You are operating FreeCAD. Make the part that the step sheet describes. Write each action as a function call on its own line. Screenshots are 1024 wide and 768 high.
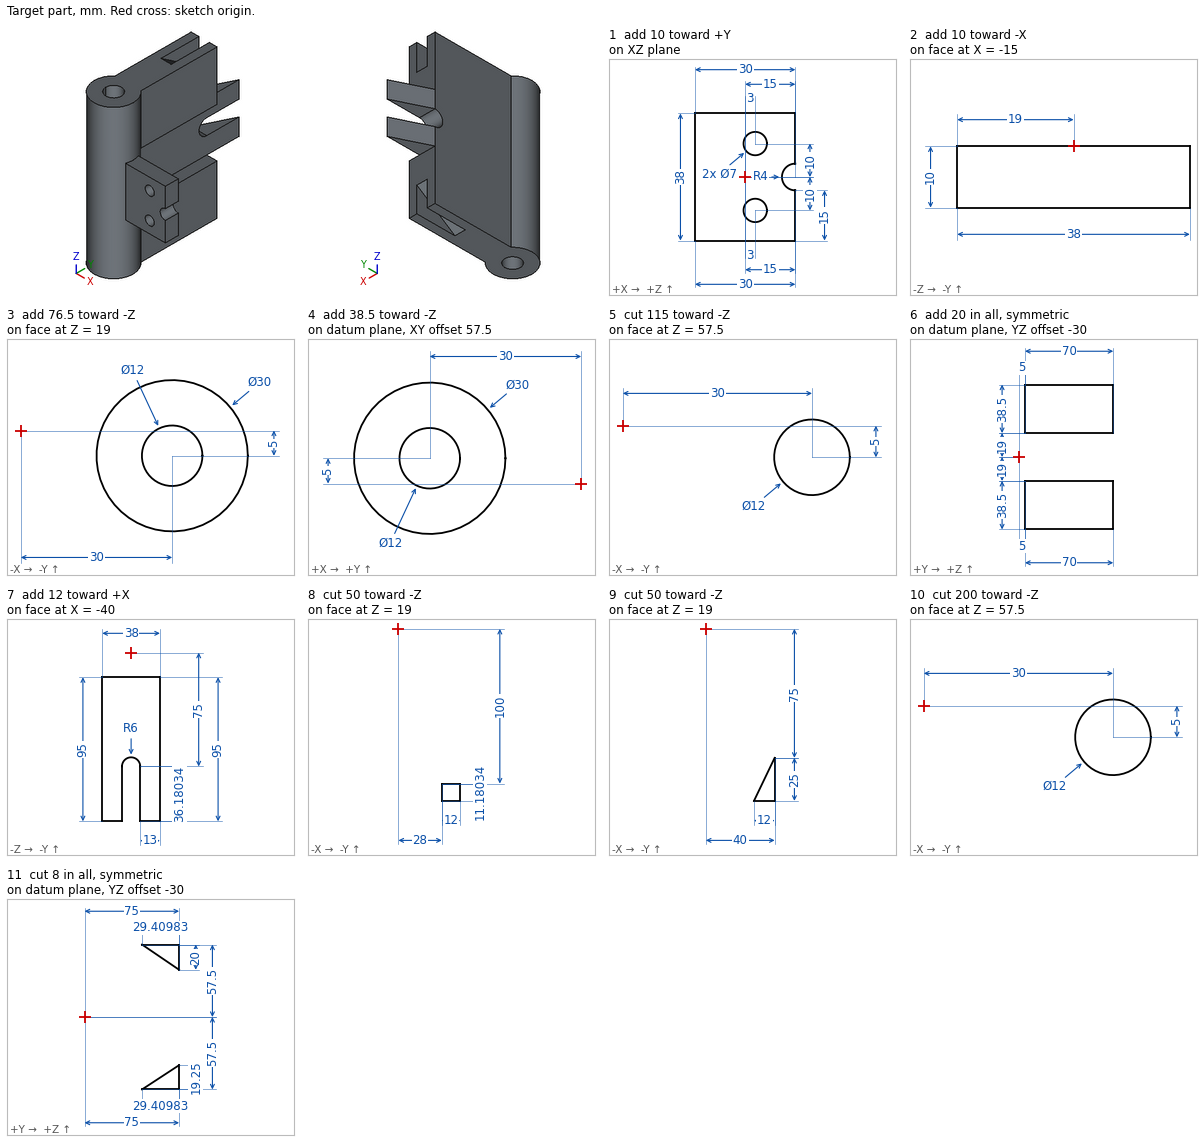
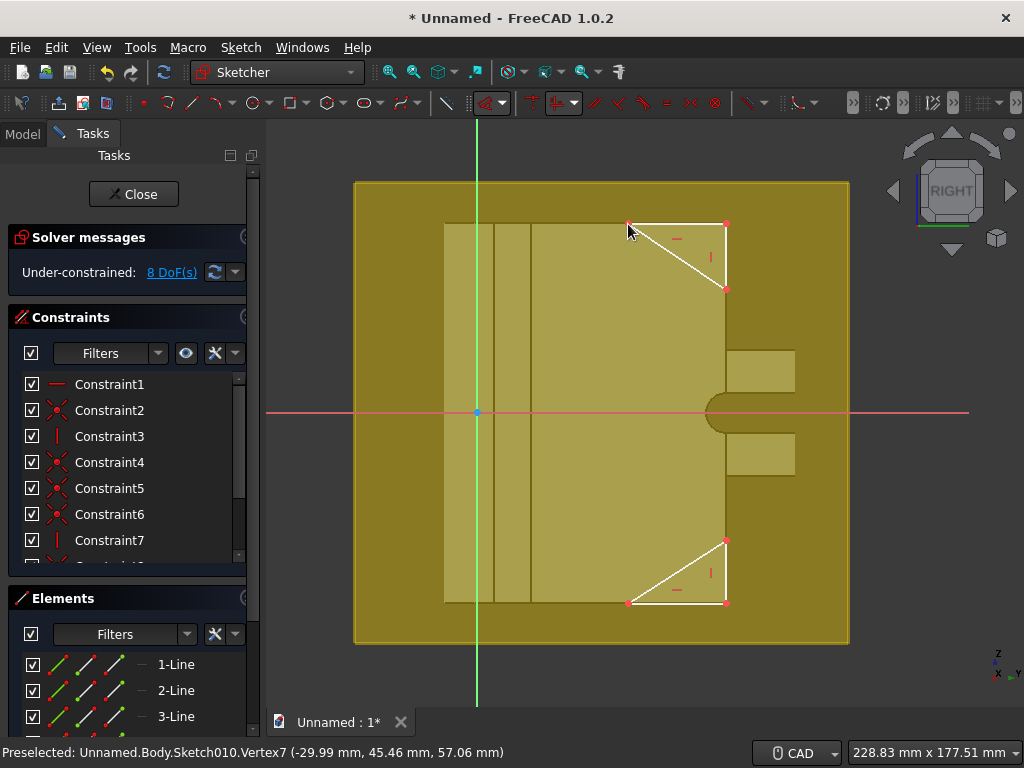
click(726, 270)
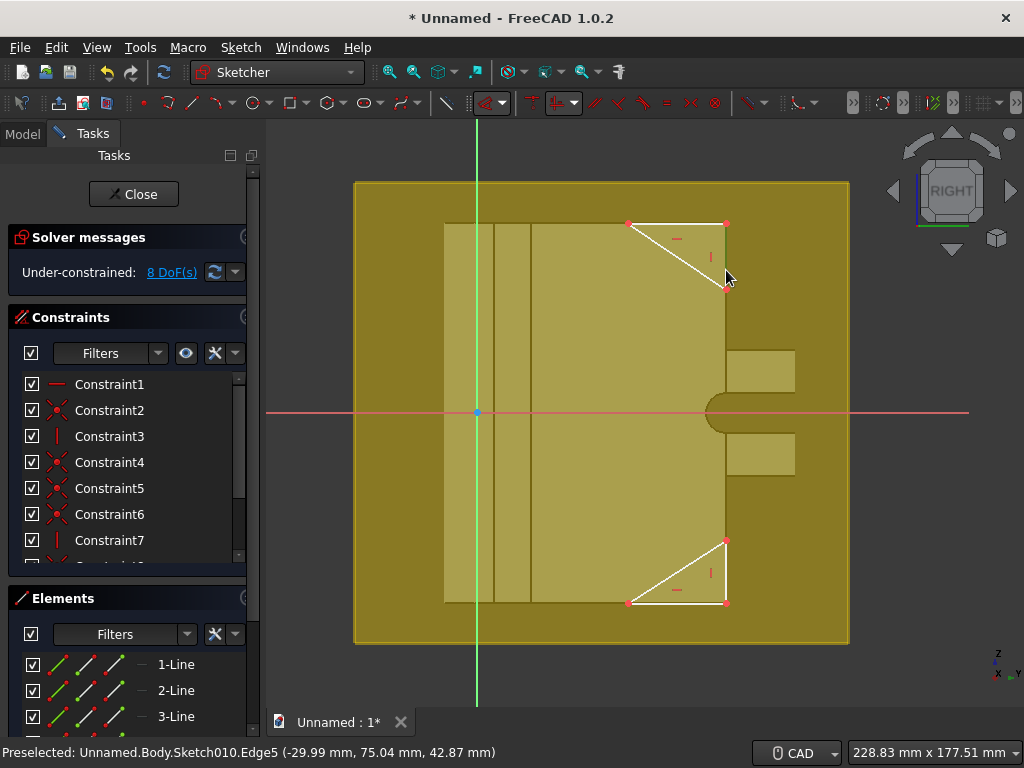
click(504, 104)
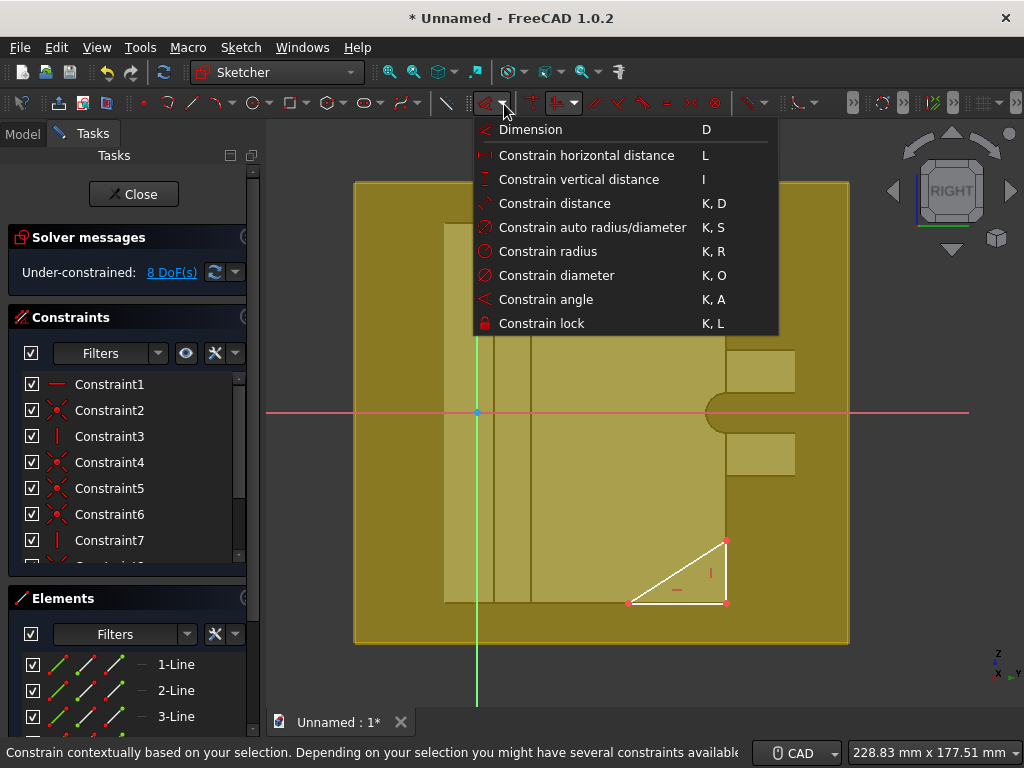
click(626, 179)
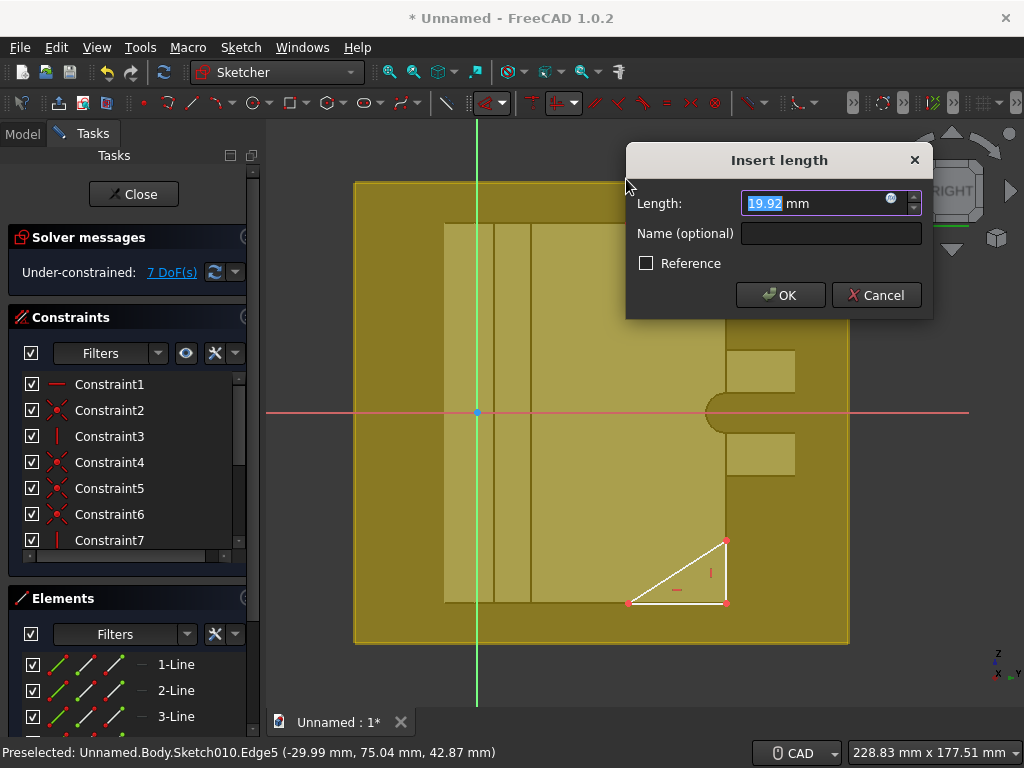
text(20)
key(Return)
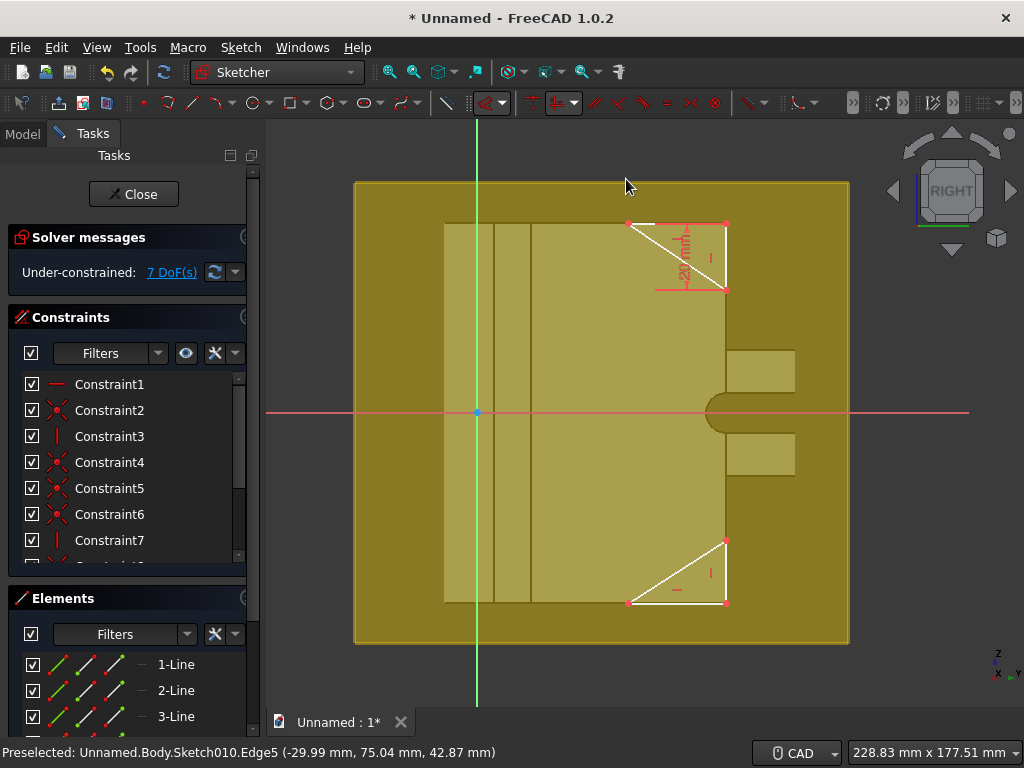
click(726, 604)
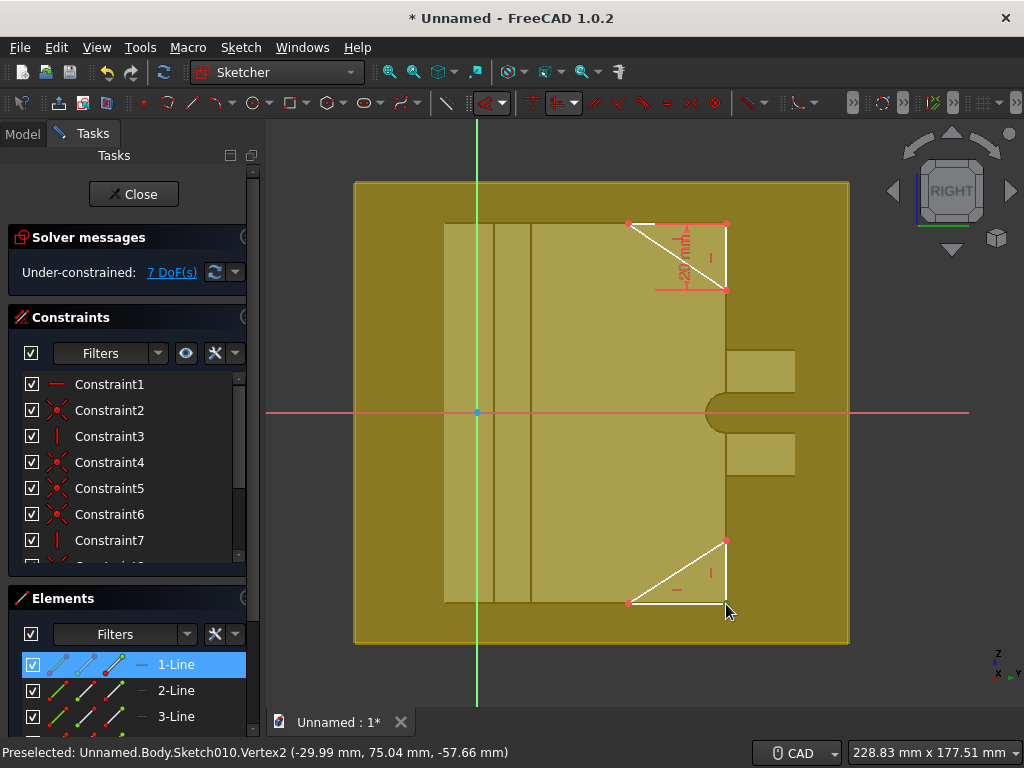
key(l)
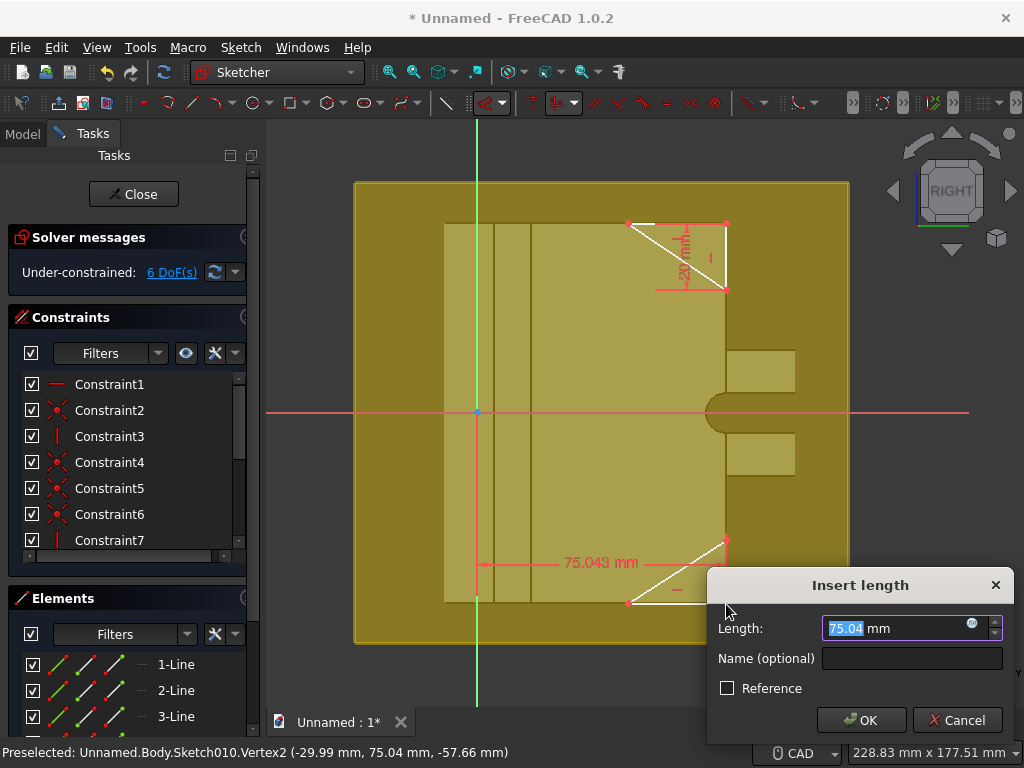
text(75)
key(Return)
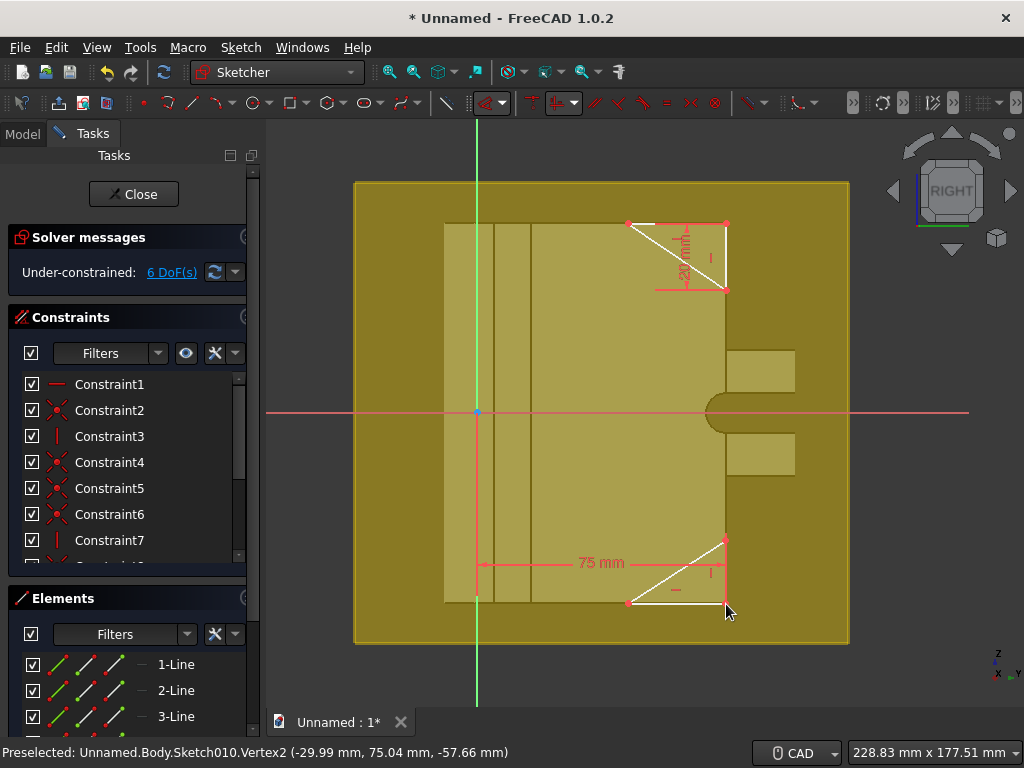
click(726, 290)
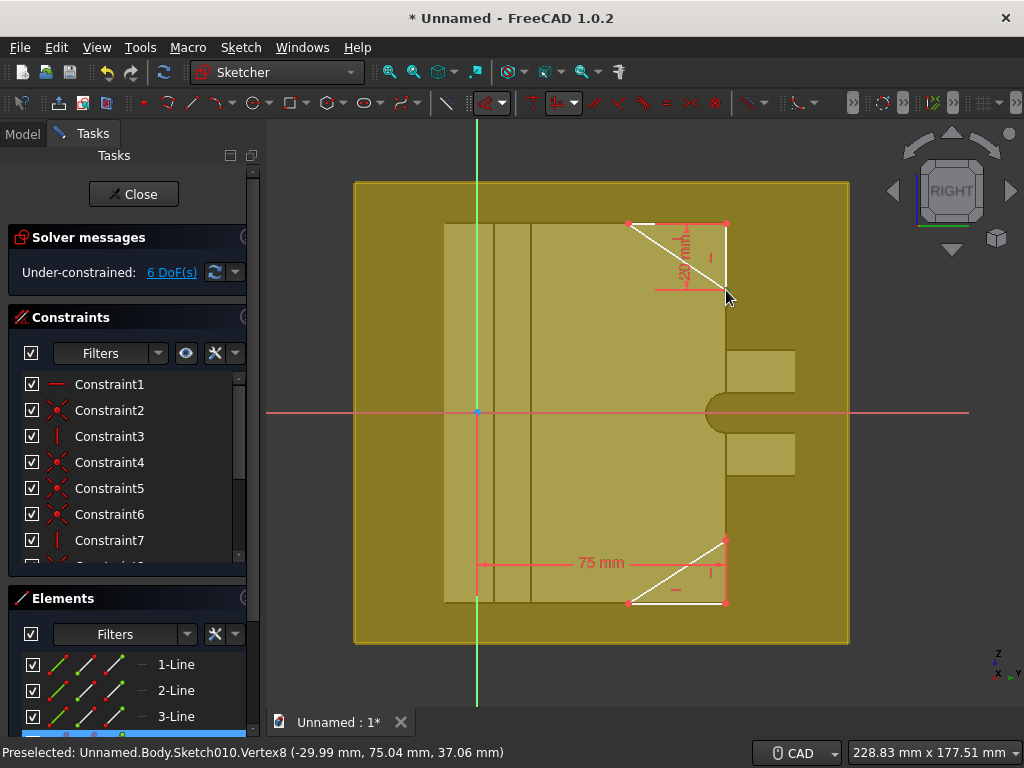
key(l)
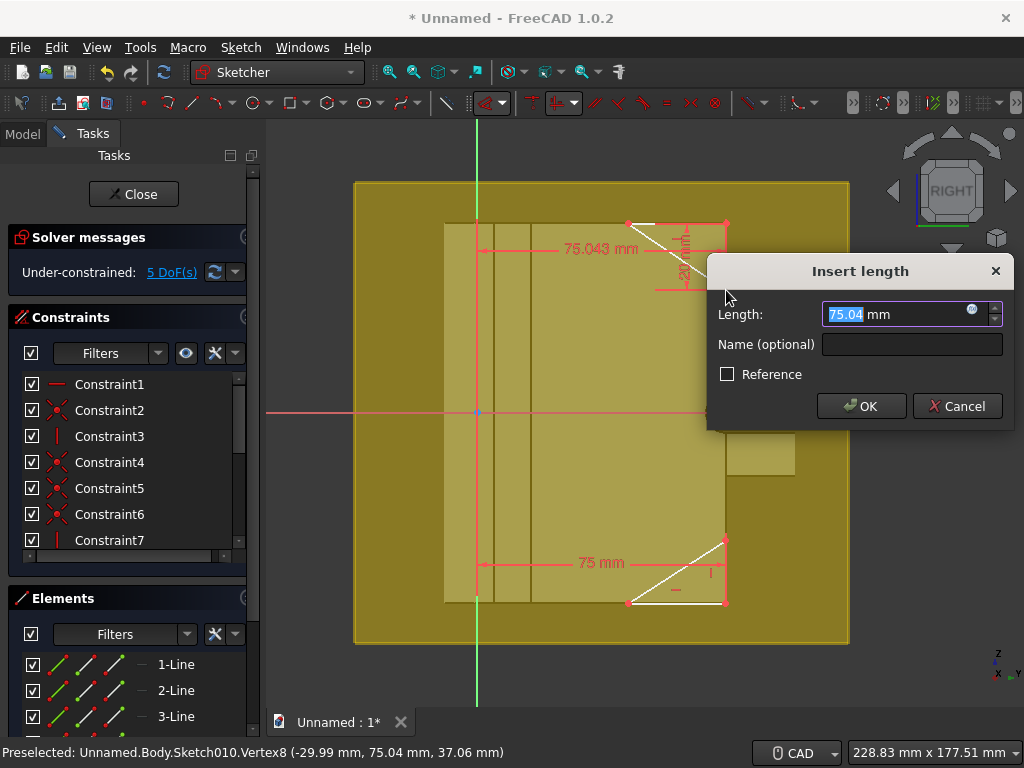
text(75)
key(Return)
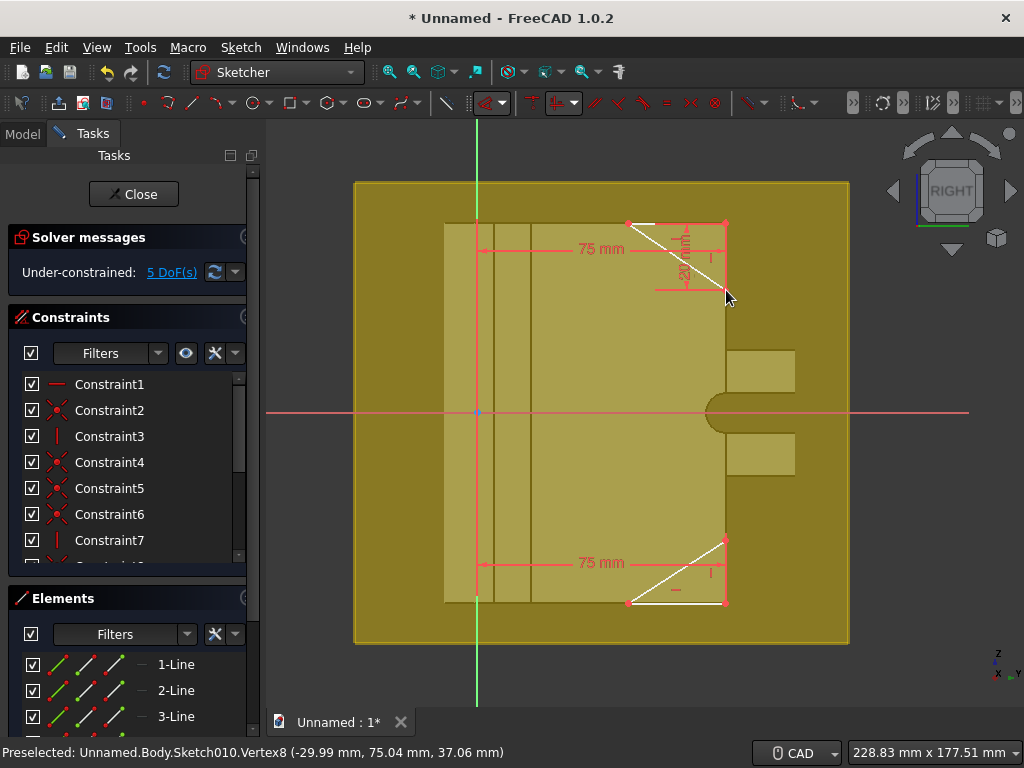
click(726, 585)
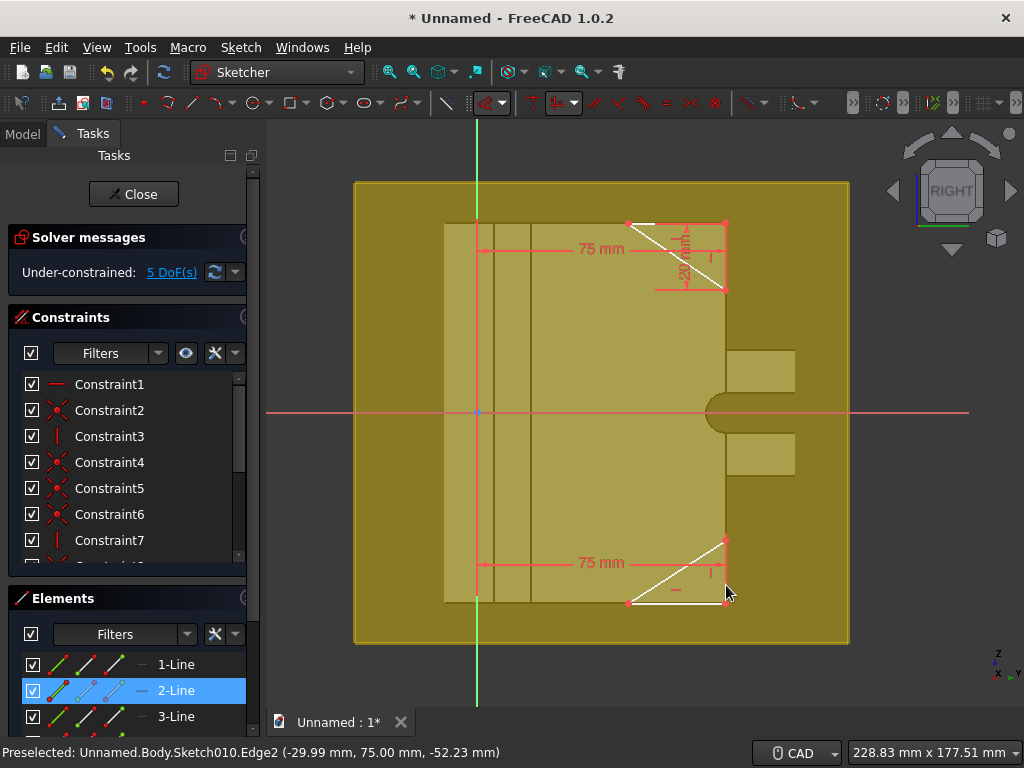
key(i)